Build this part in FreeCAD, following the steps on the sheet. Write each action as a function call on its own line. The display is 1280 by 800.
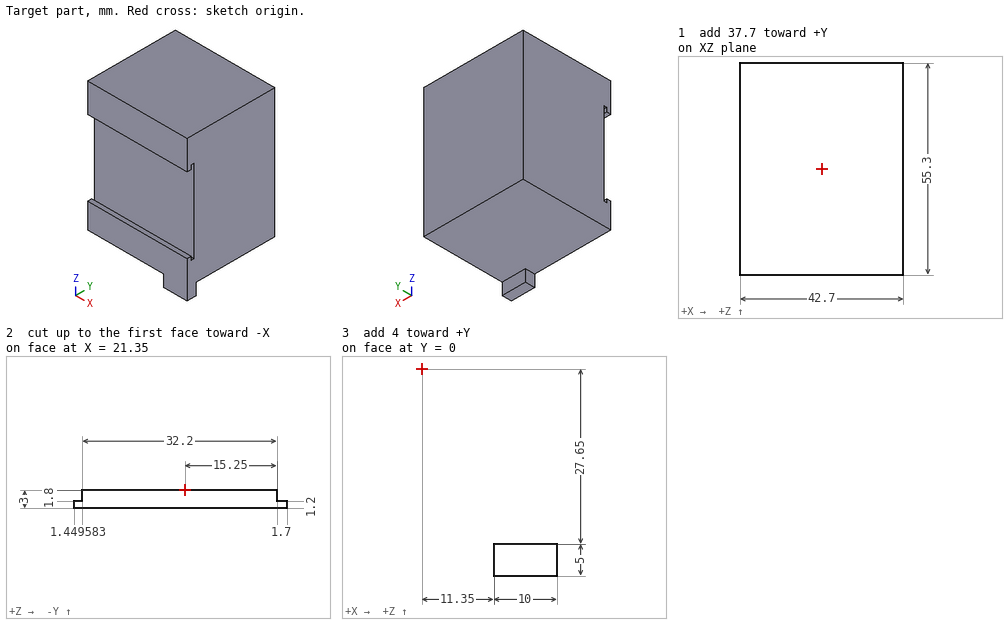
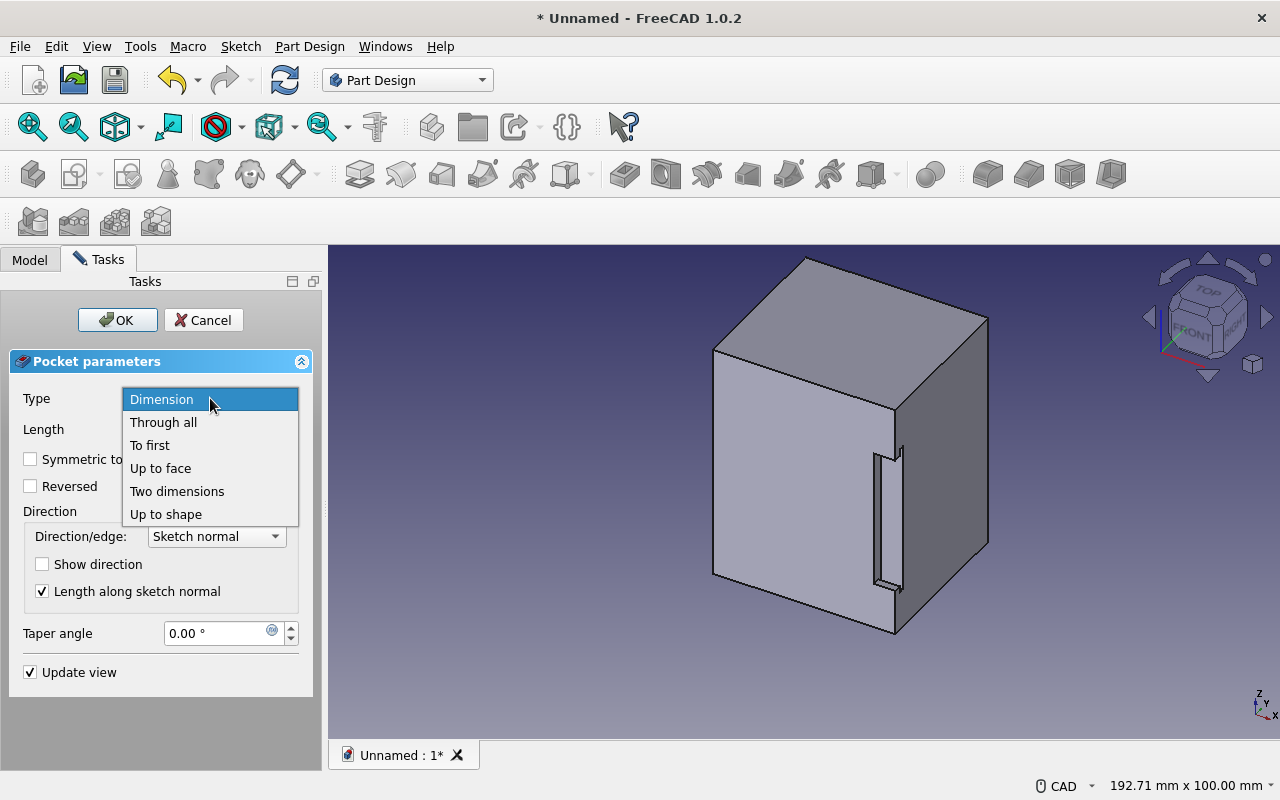
click(208, 446)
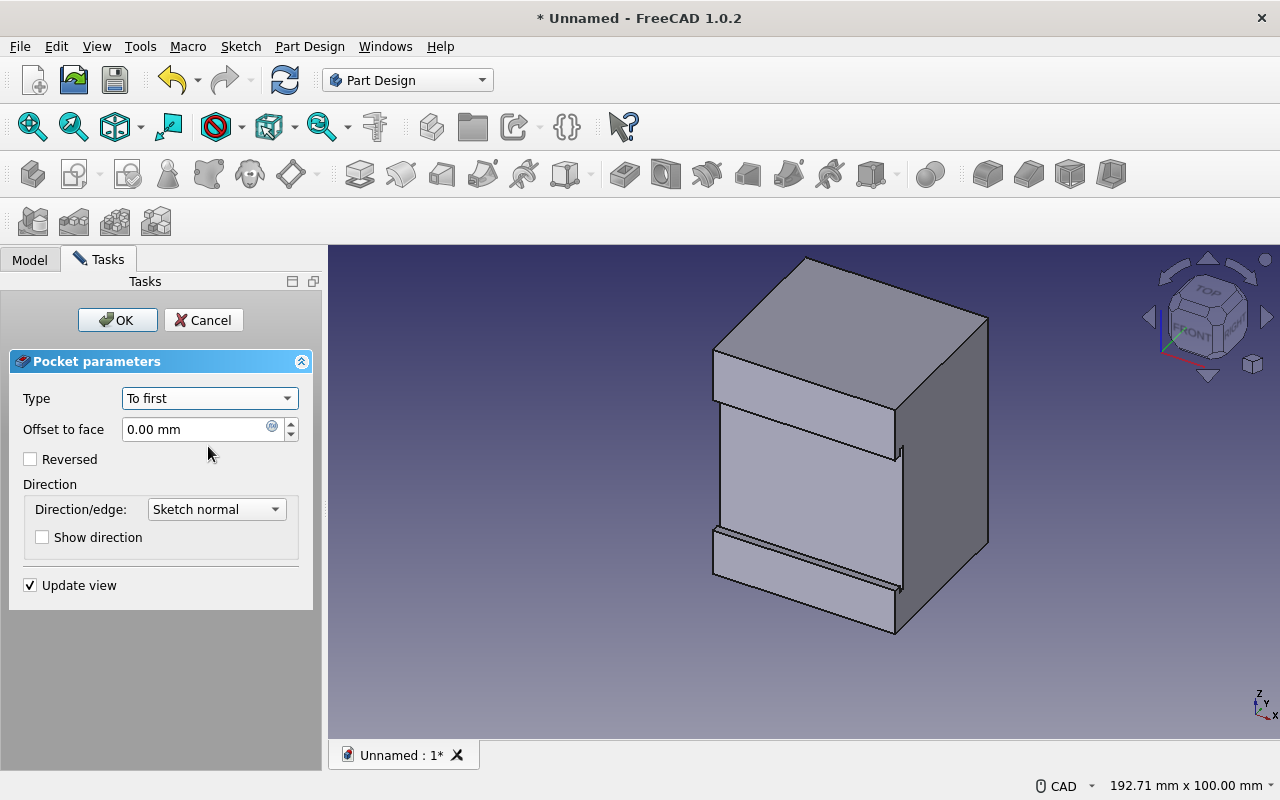
click(118, 320)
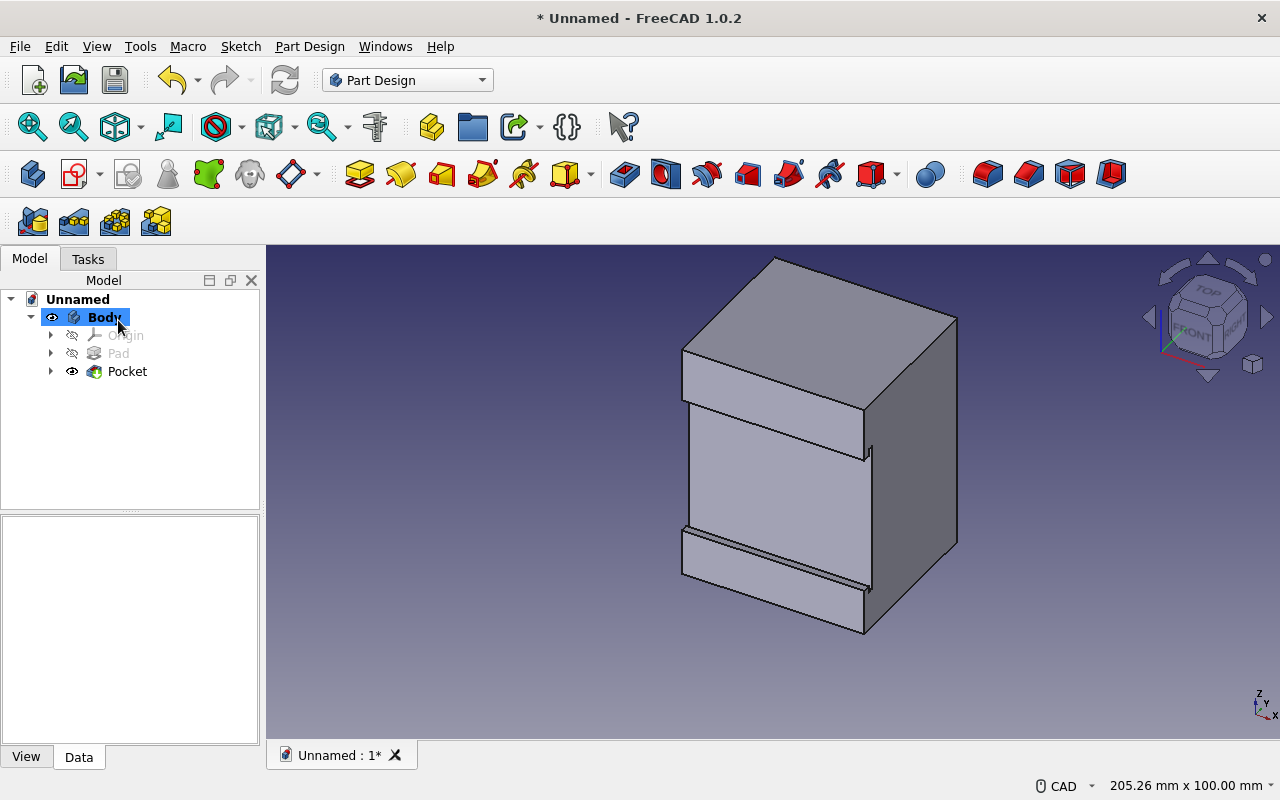
click(825, 421)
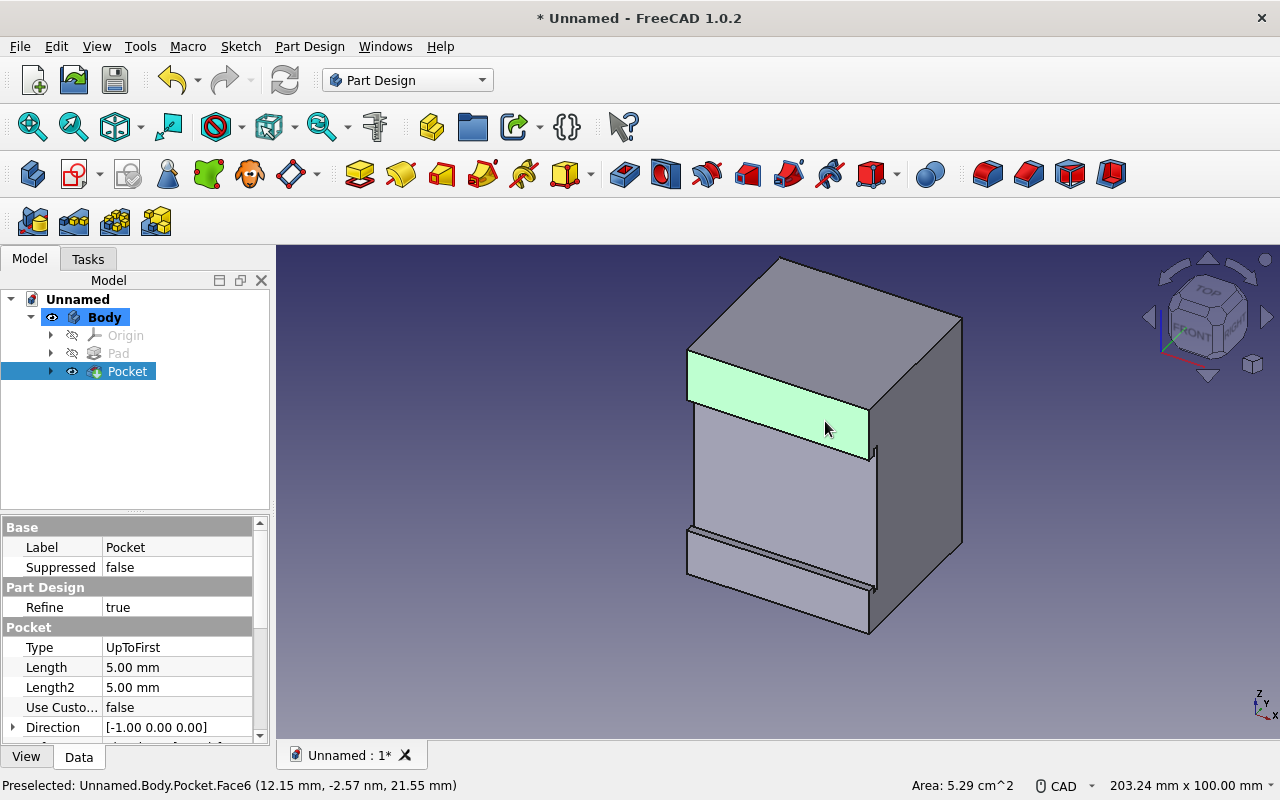
click(74, 174)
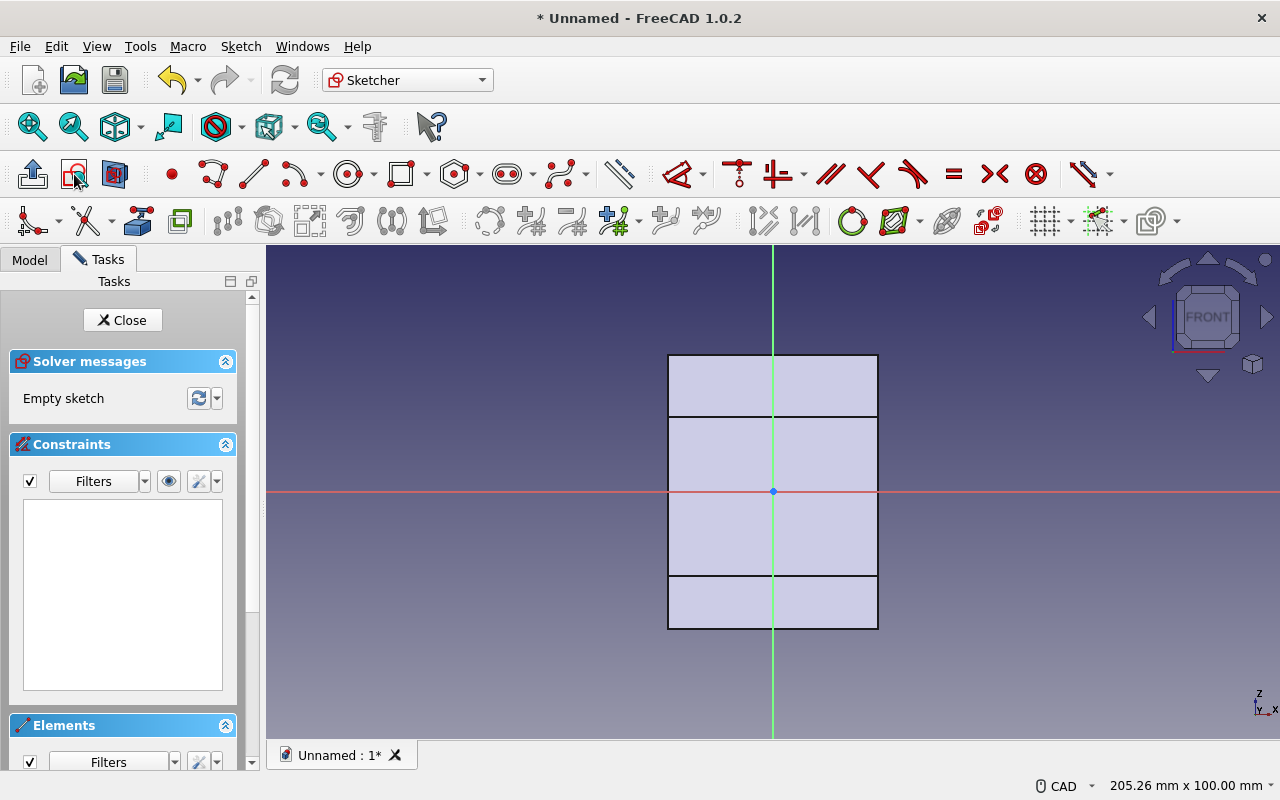
scroll(869, 656, up, 12)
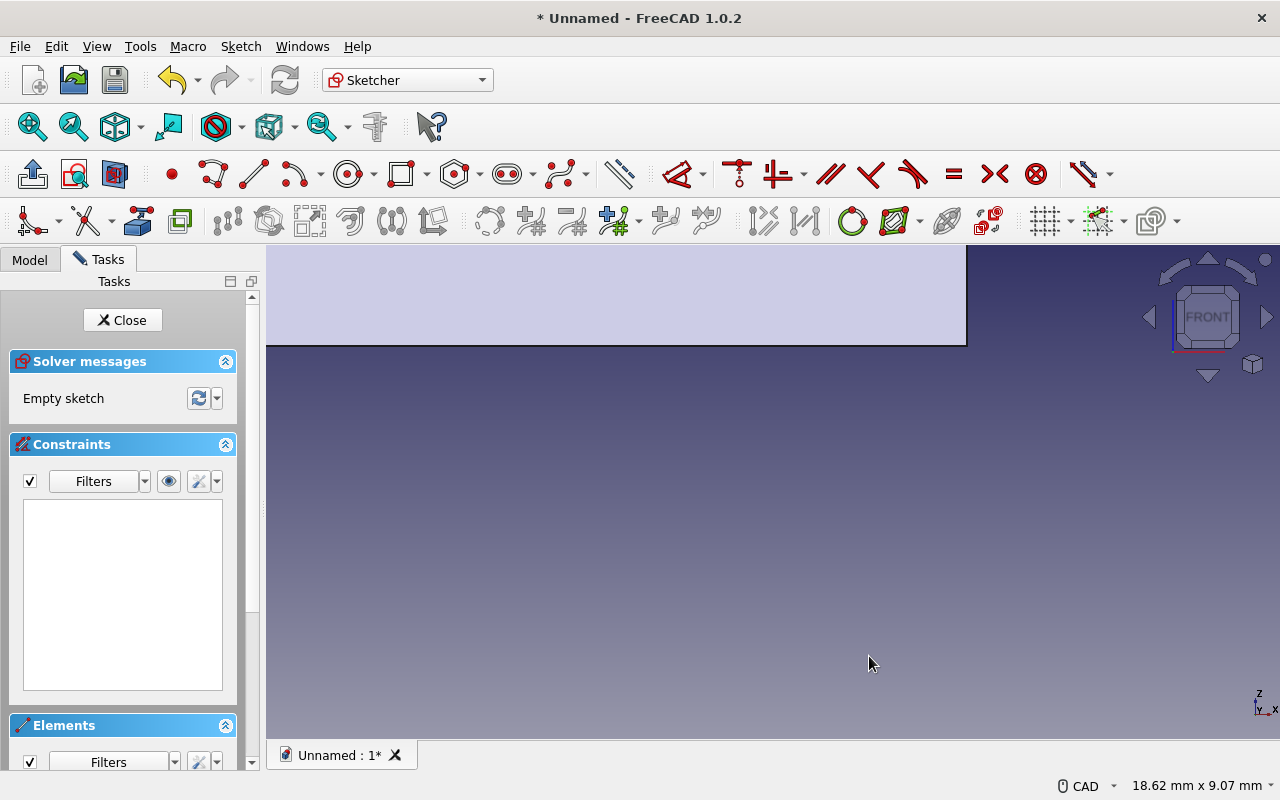
key(g)
key(r)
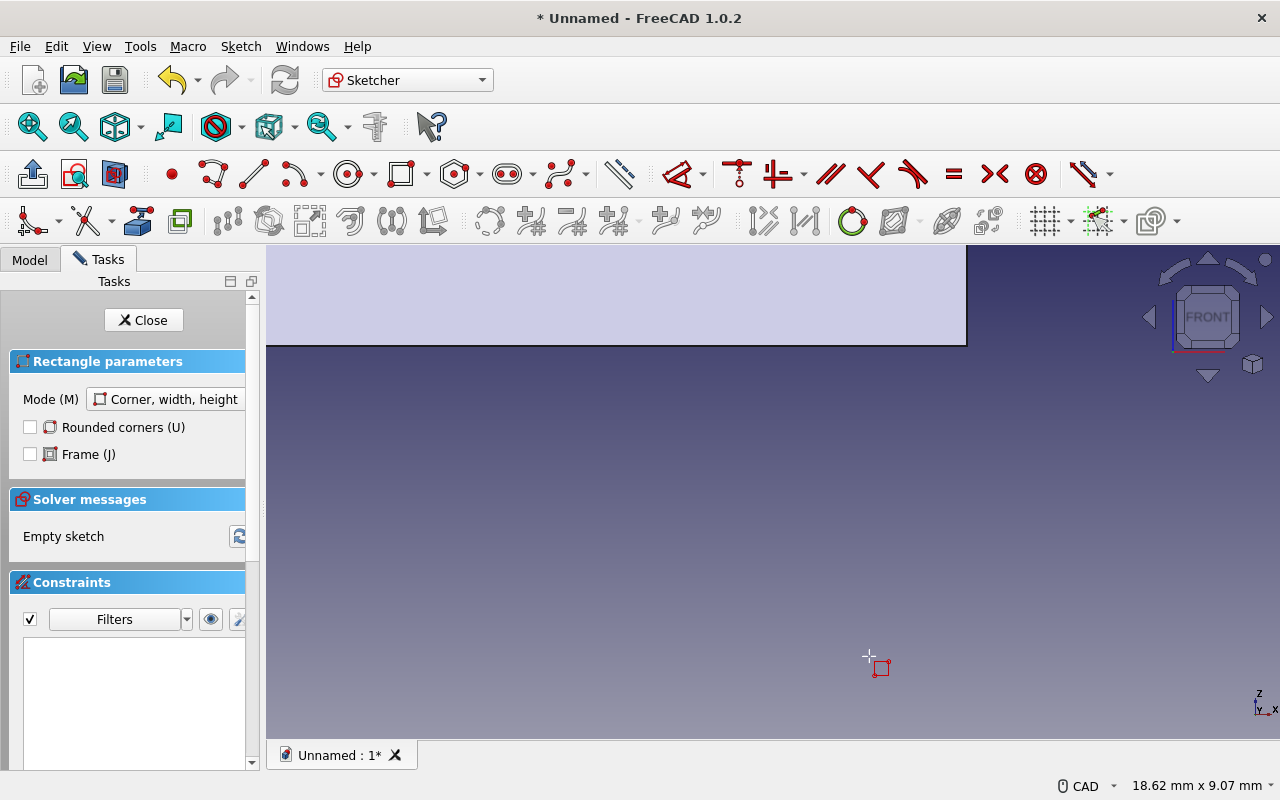
click(423, 346)
move(967, 618)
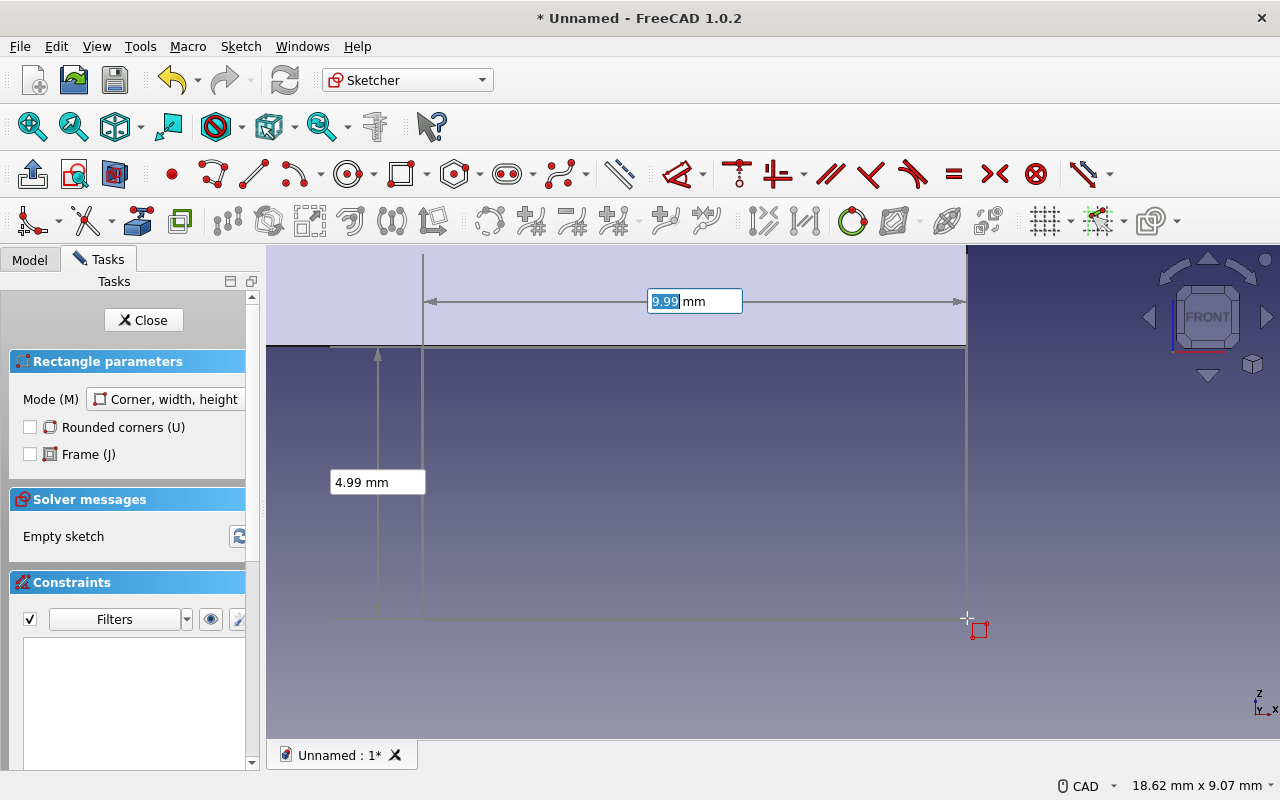
text(10)
key(Tab)
text(5)
key(Return)
key(Escape)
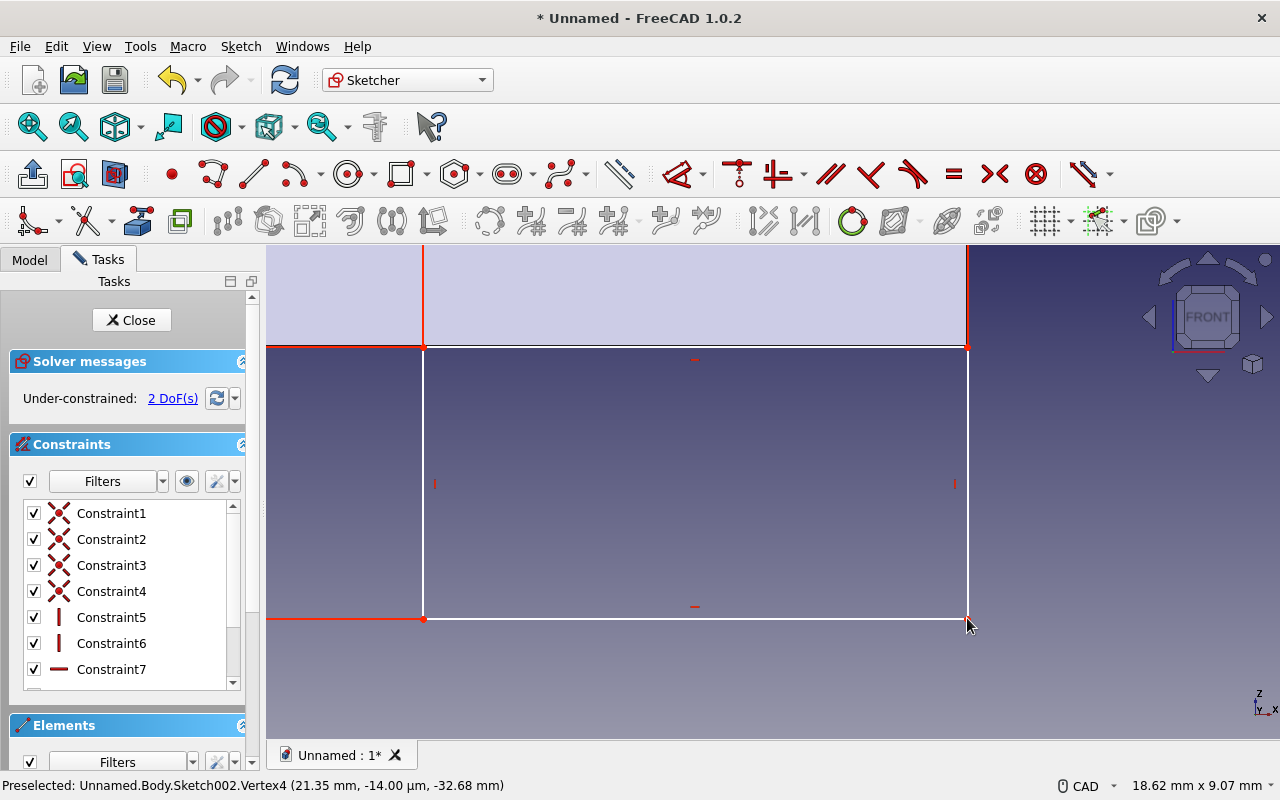
key(d)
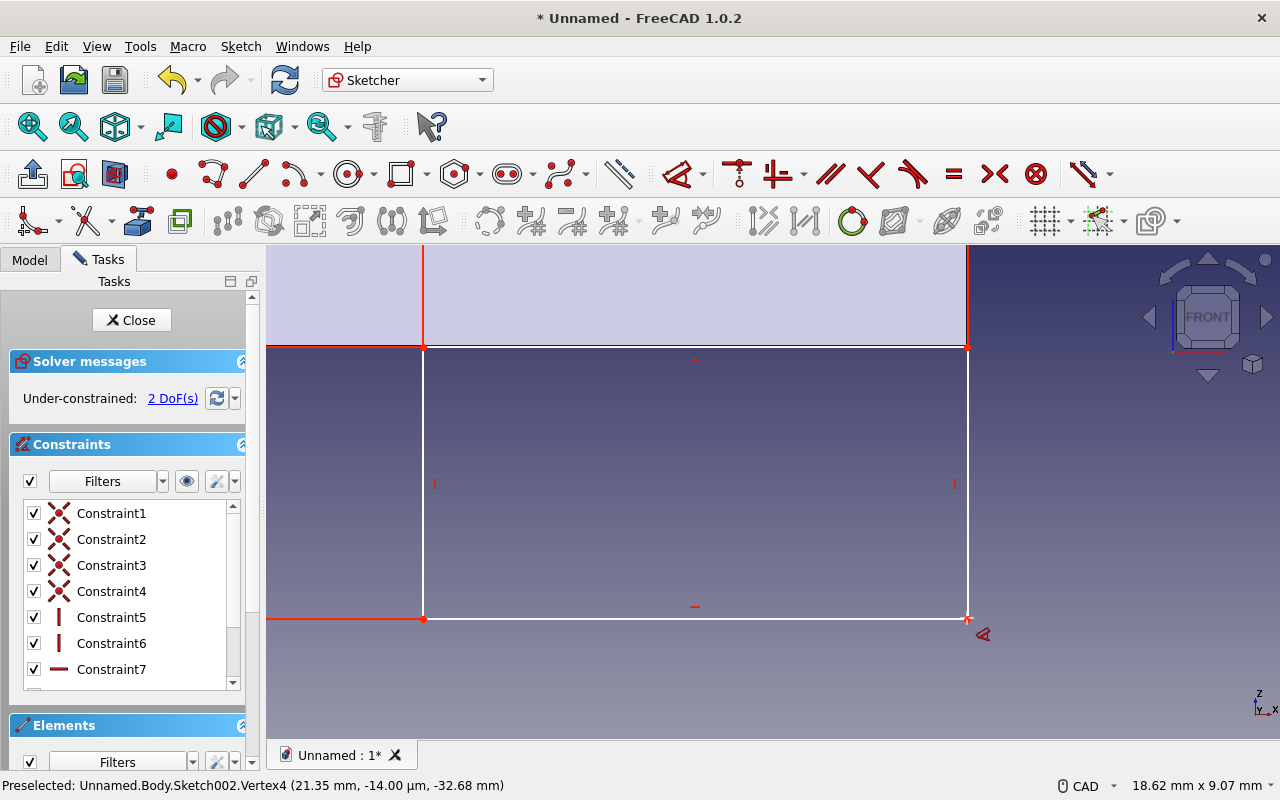
click(423, 347)
click(359, 381)